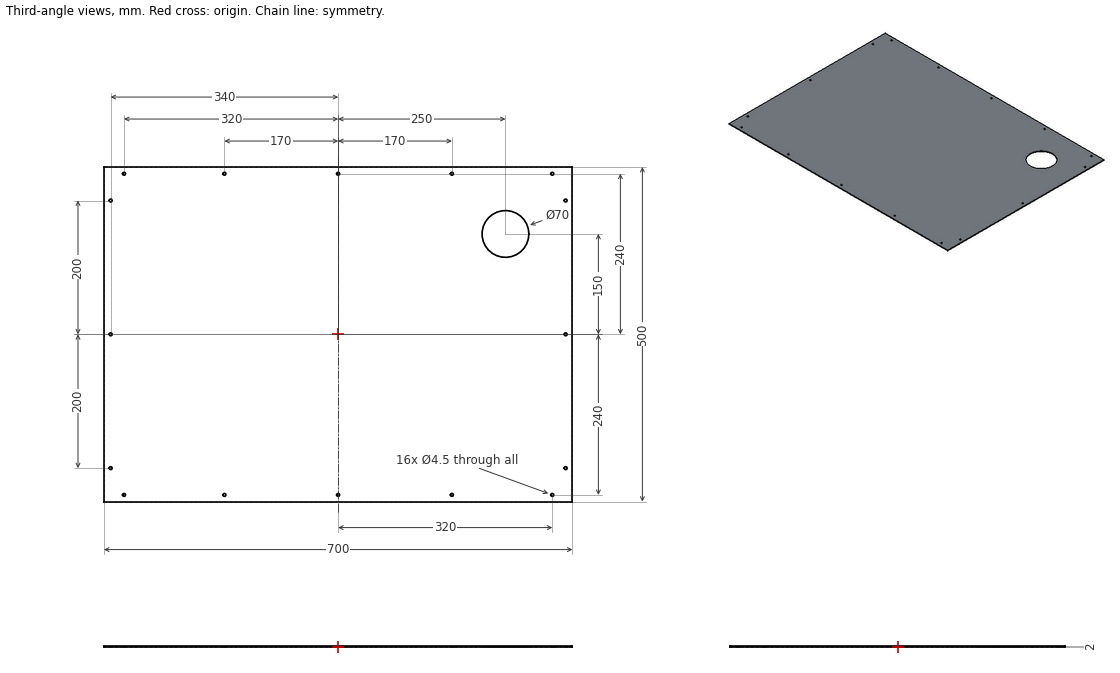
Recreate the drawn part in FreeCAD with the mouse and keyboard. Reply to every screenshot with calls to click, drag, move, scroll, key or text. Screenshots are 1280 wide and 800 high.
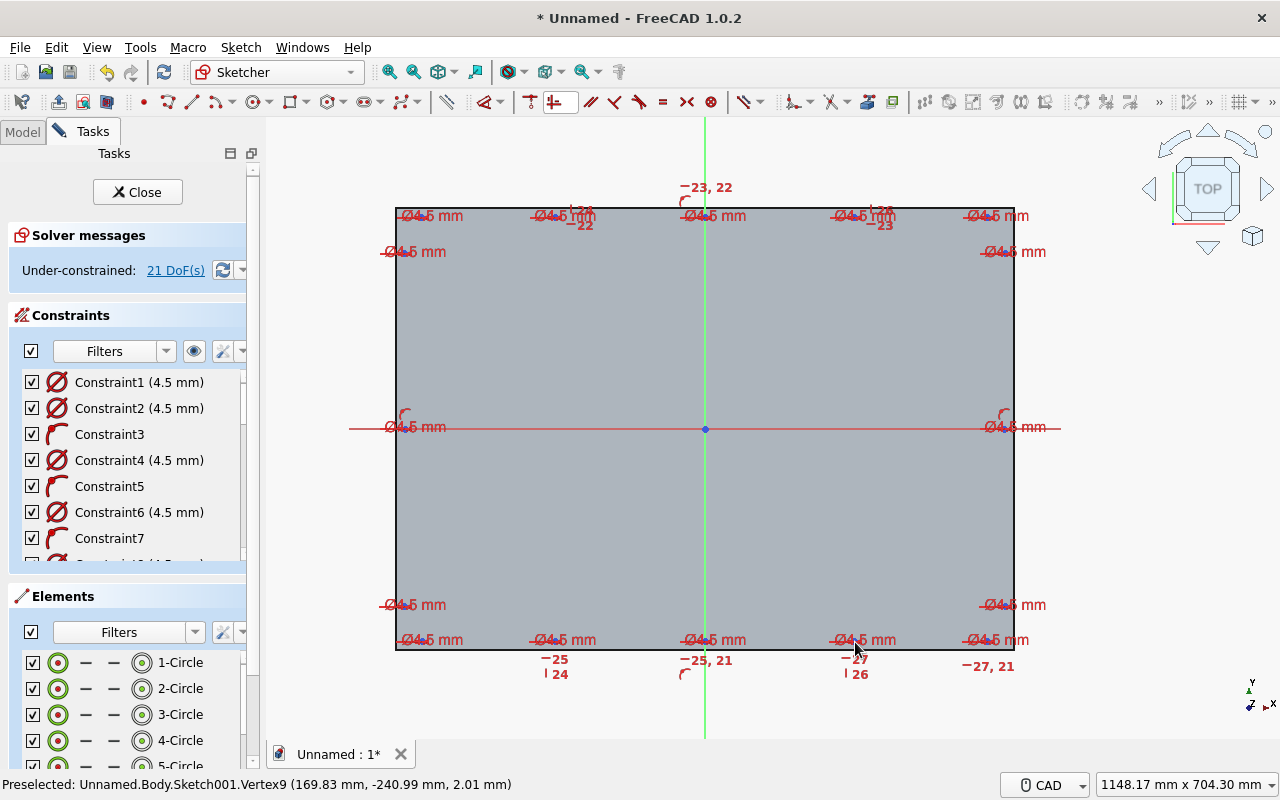
click(555, 218)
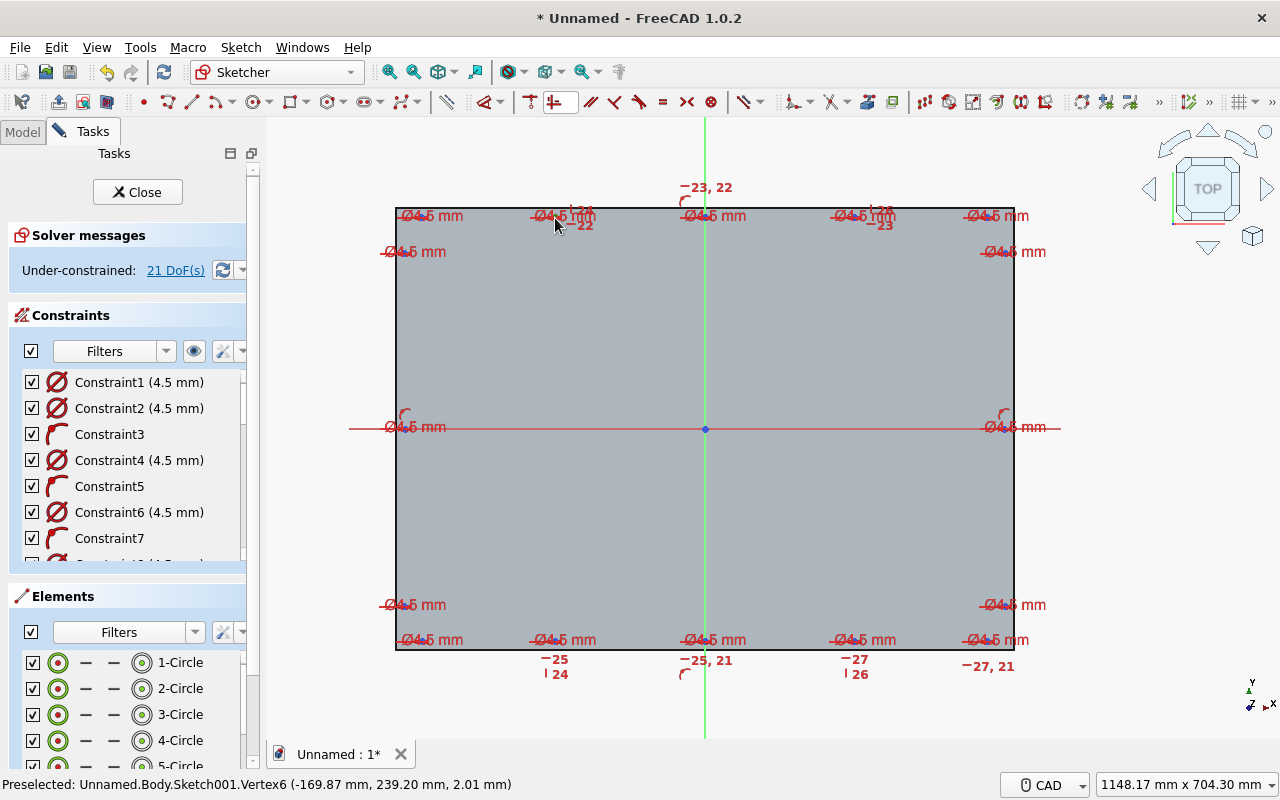
click(422, 218)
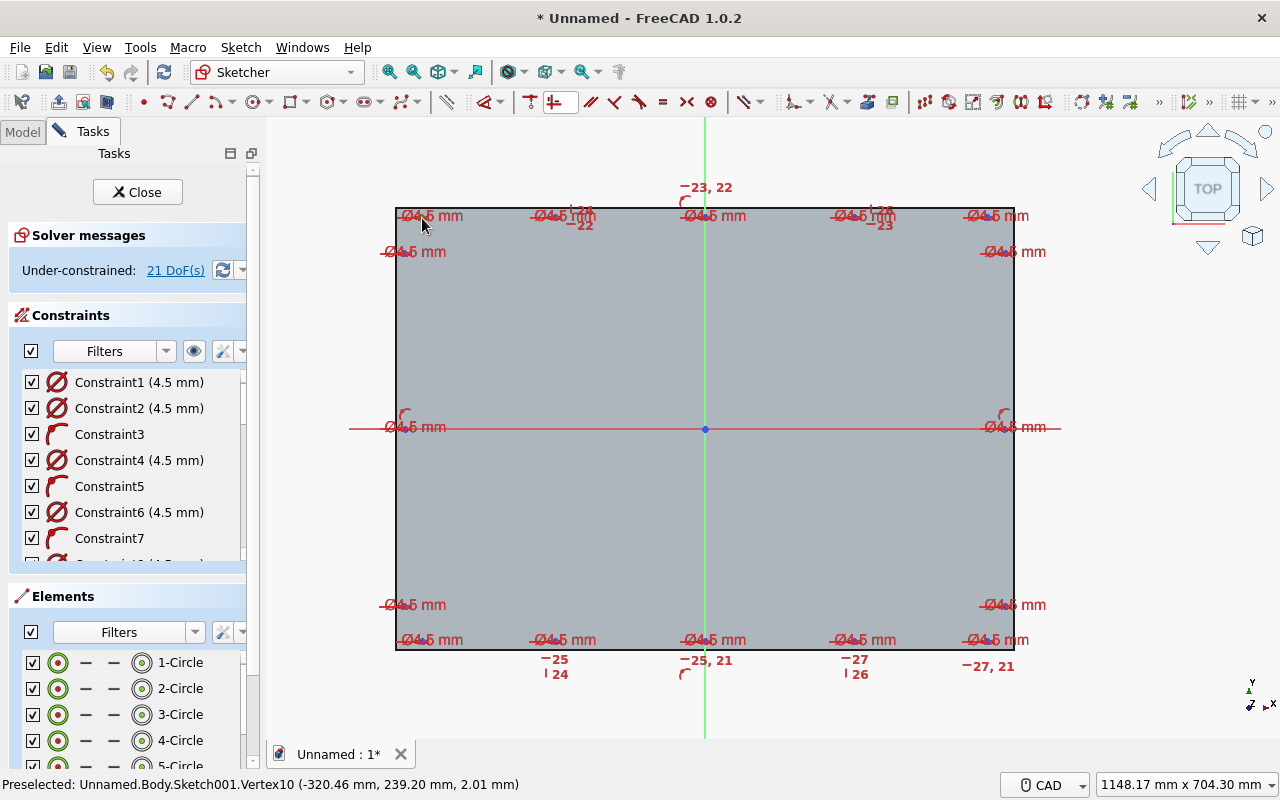
key(h)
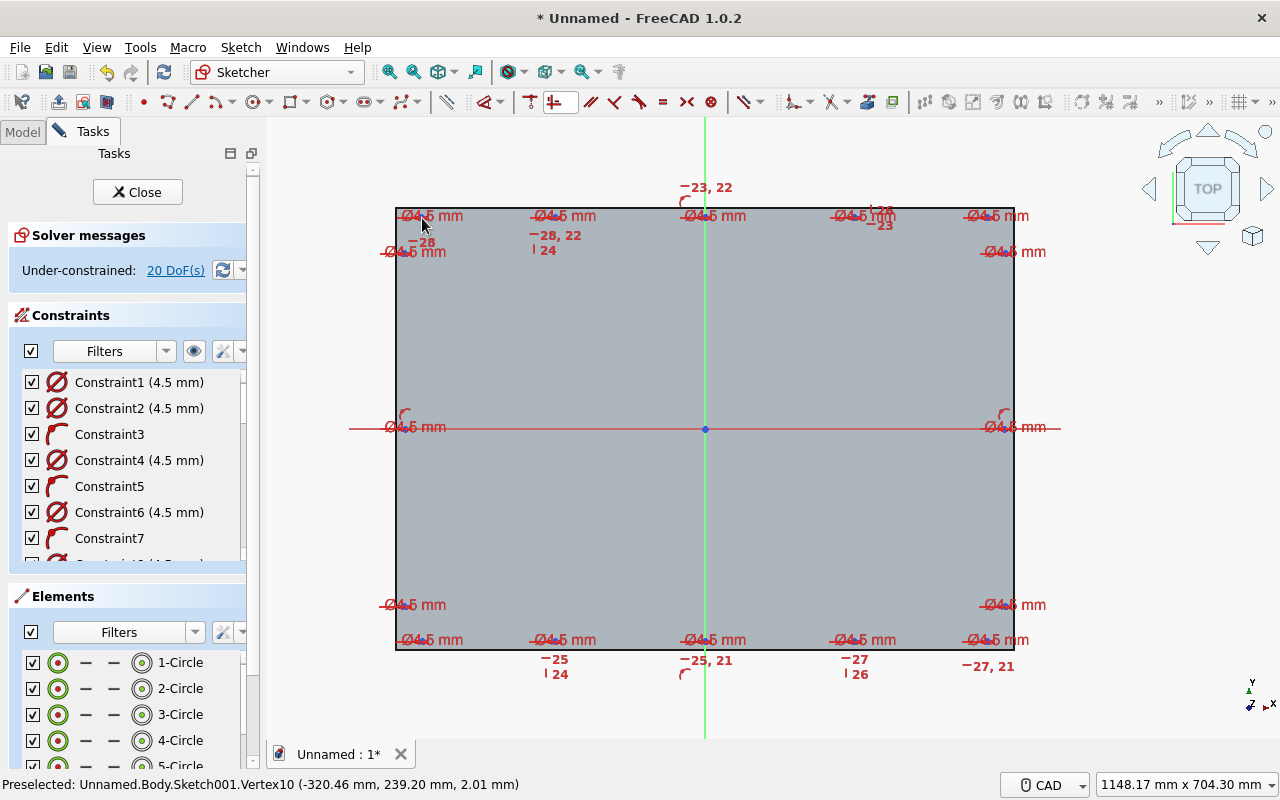
click(988, 642)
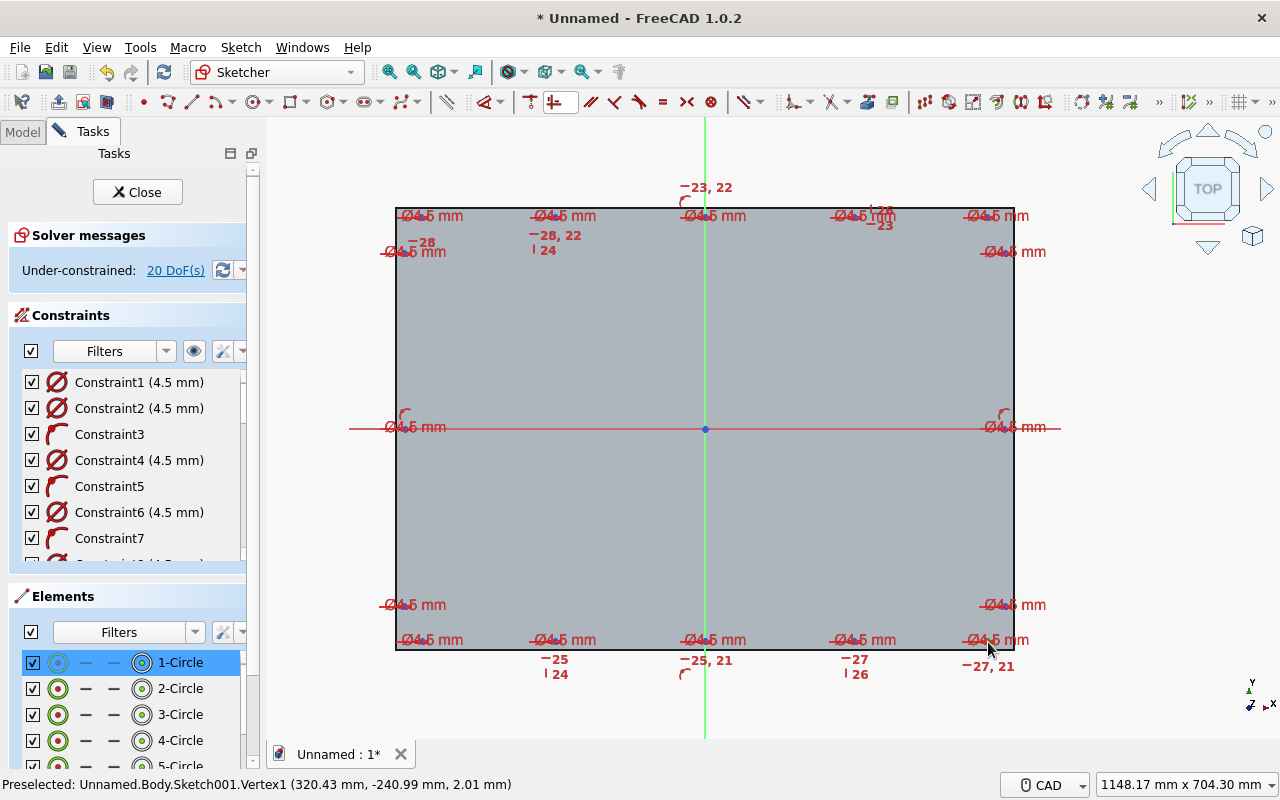
click(988, 218)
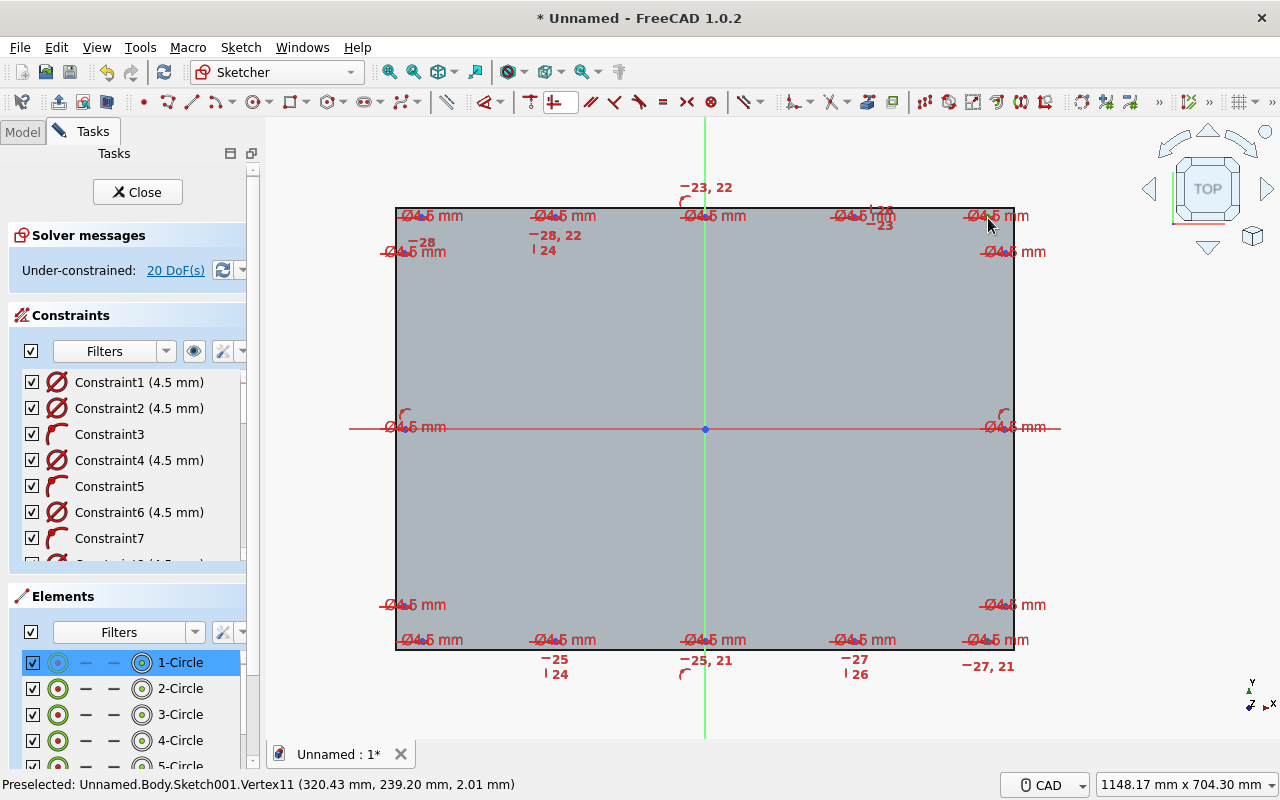
key(v)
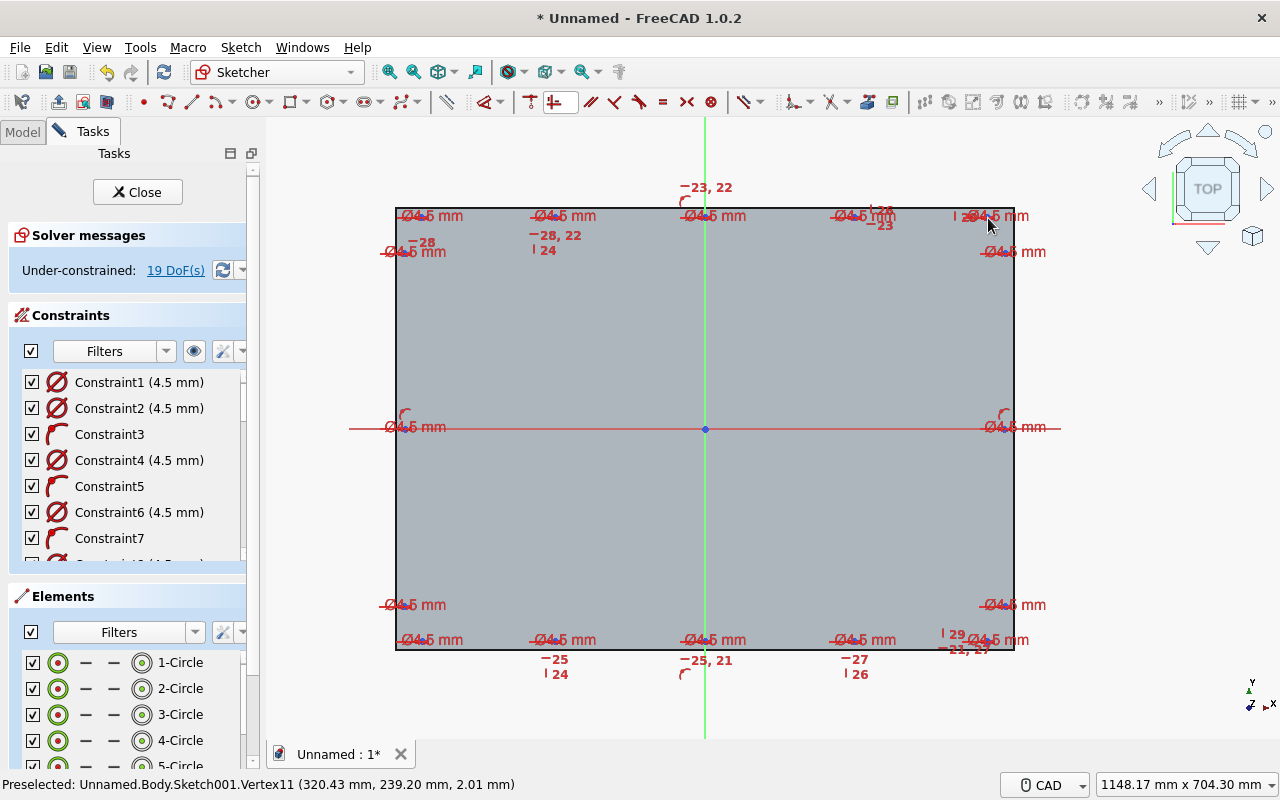
click(855, 218)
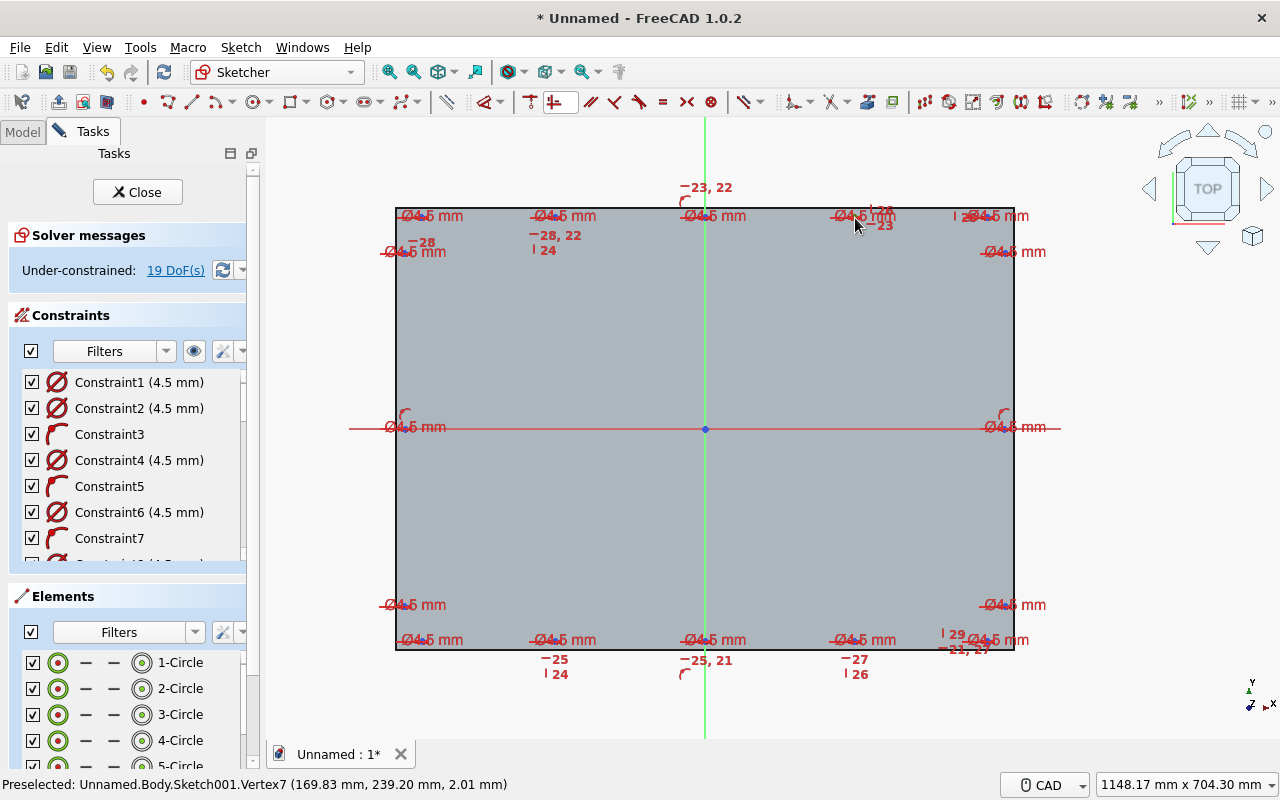
click(988, 218)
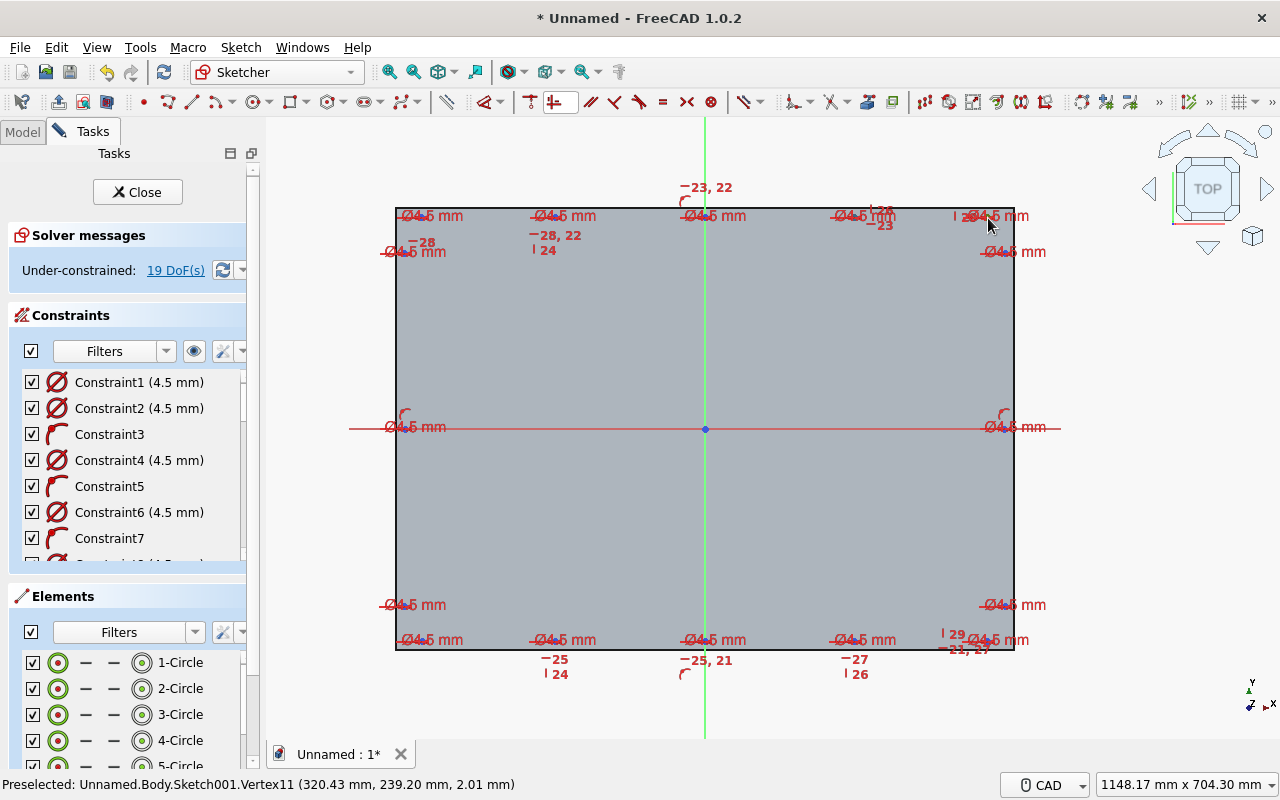
key(h)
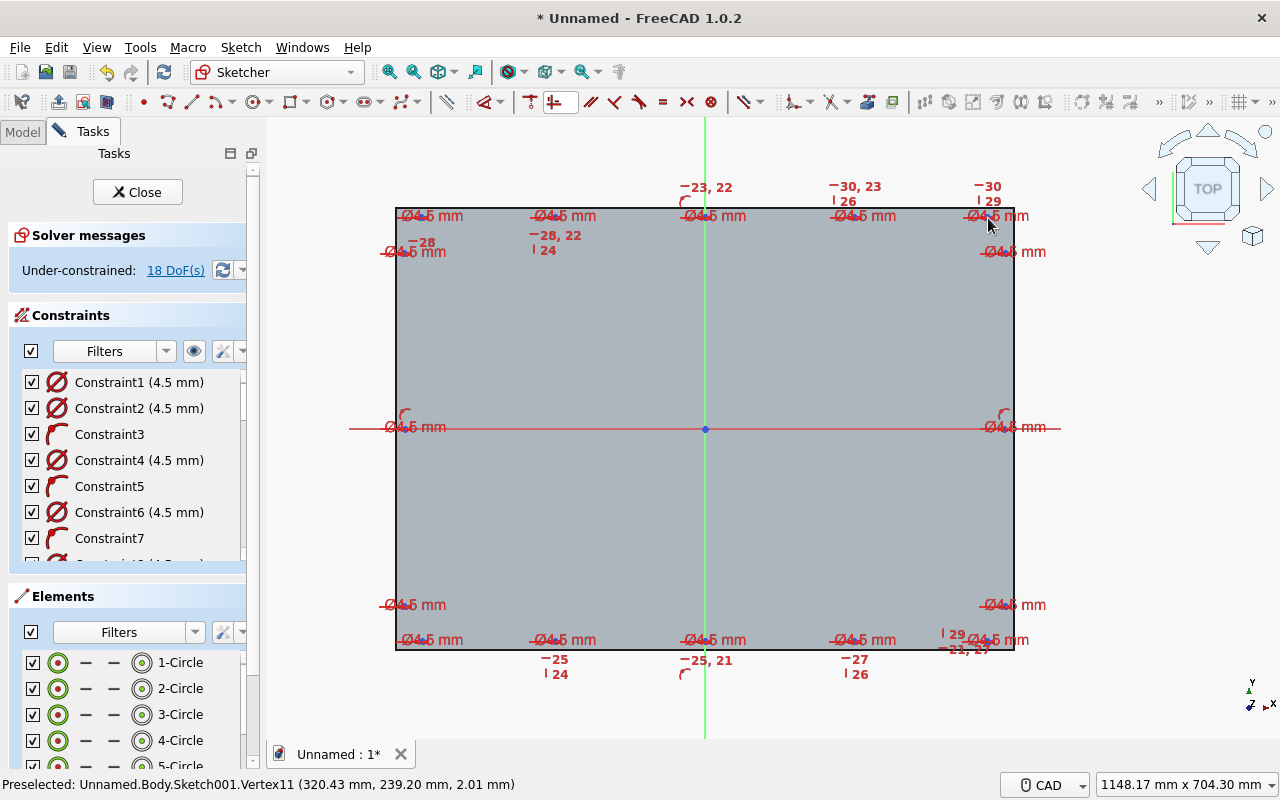
click(405, 429)